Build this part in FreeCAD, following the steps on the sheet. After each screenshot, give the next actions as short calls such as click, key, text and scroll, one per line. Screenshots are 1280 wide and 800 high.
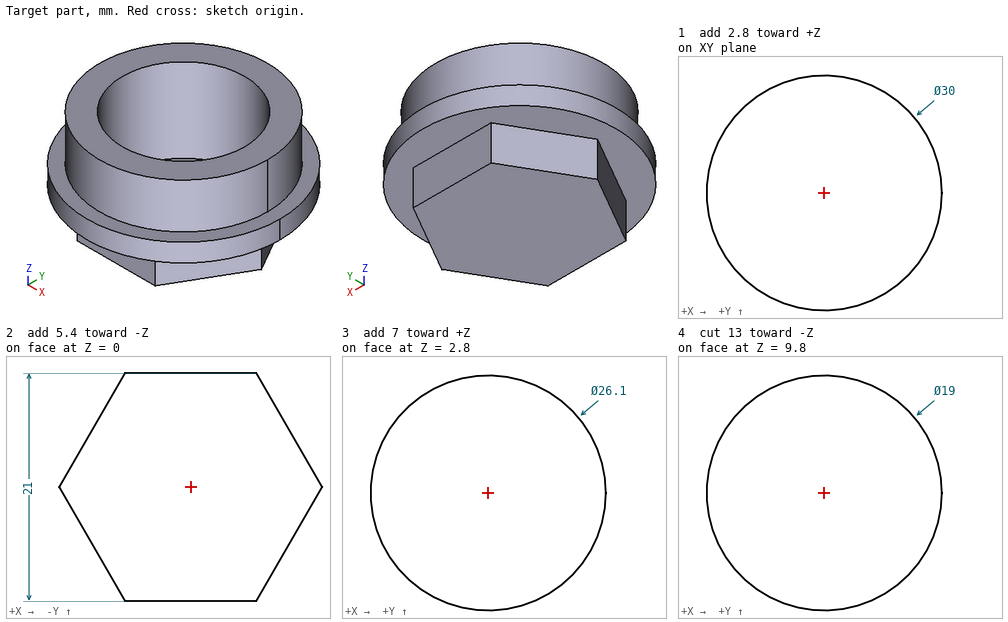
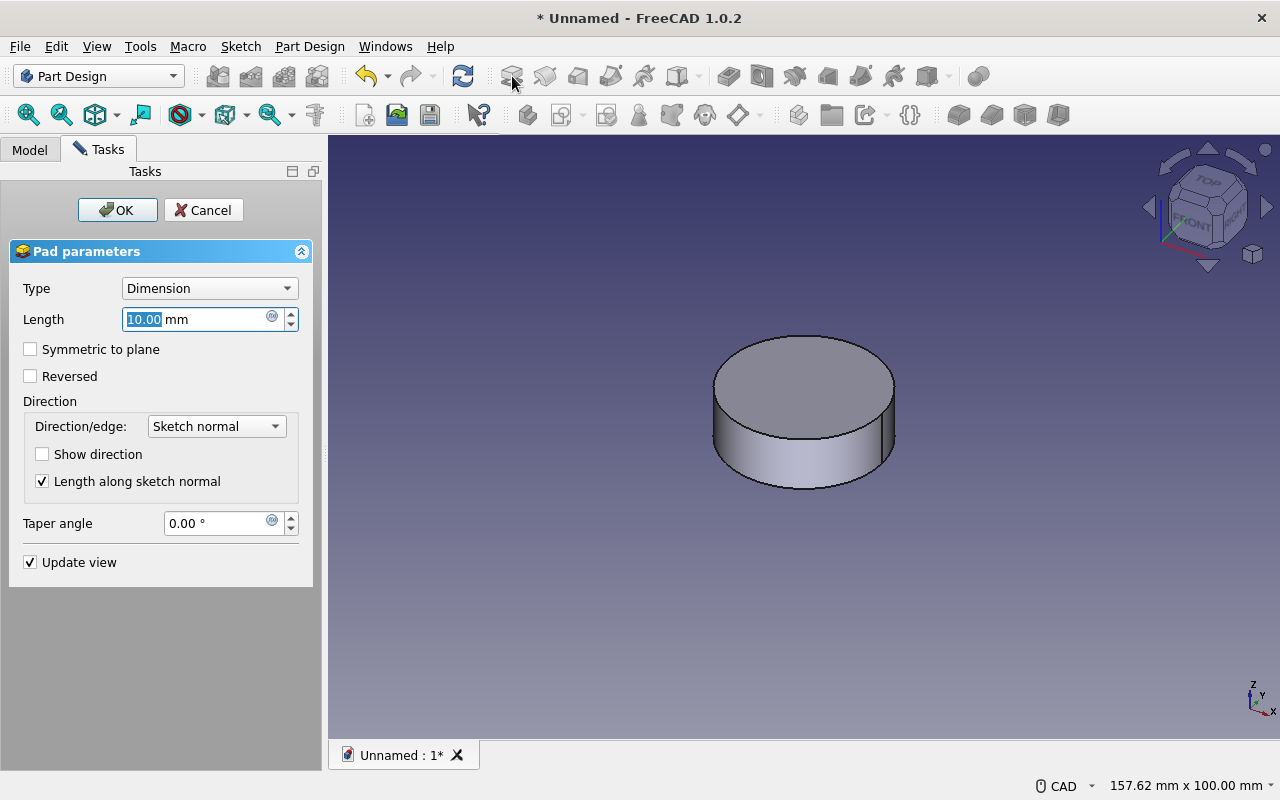
text(2.8)
key(Tab)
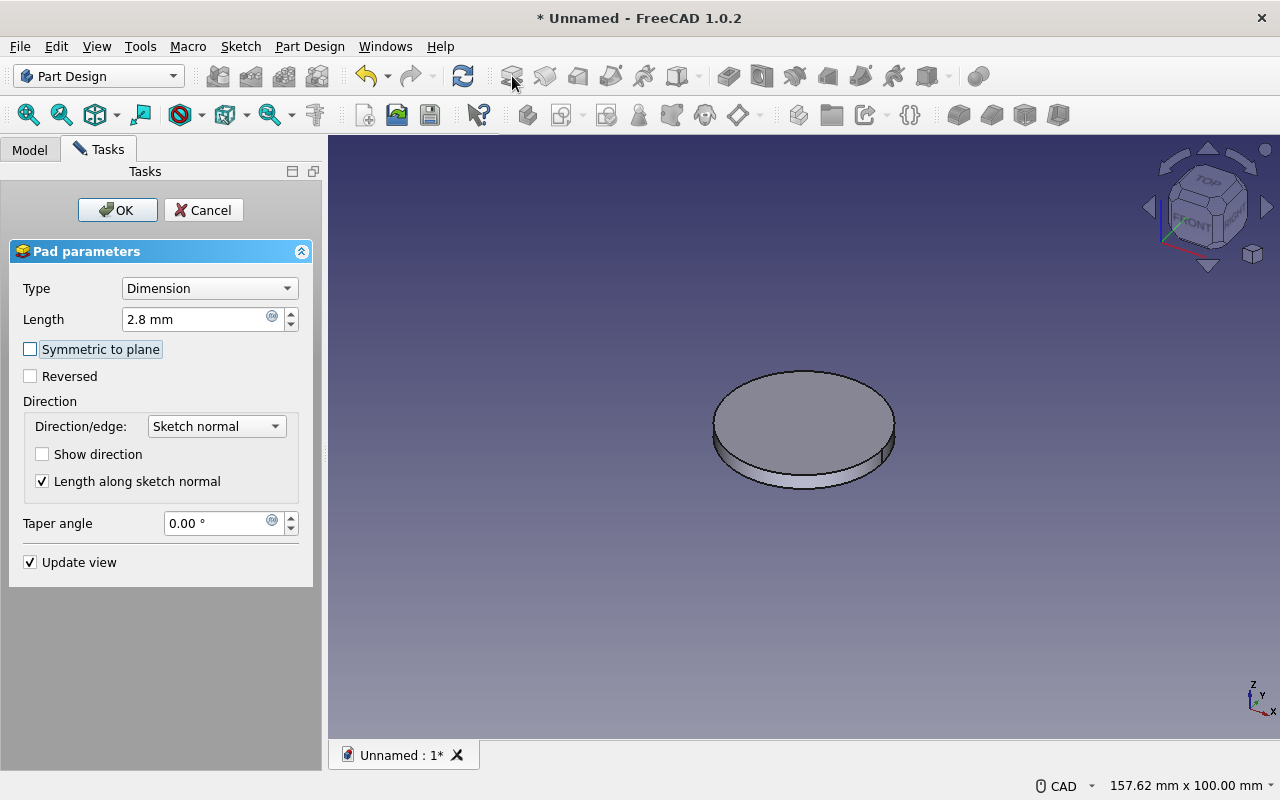
click(118, 210)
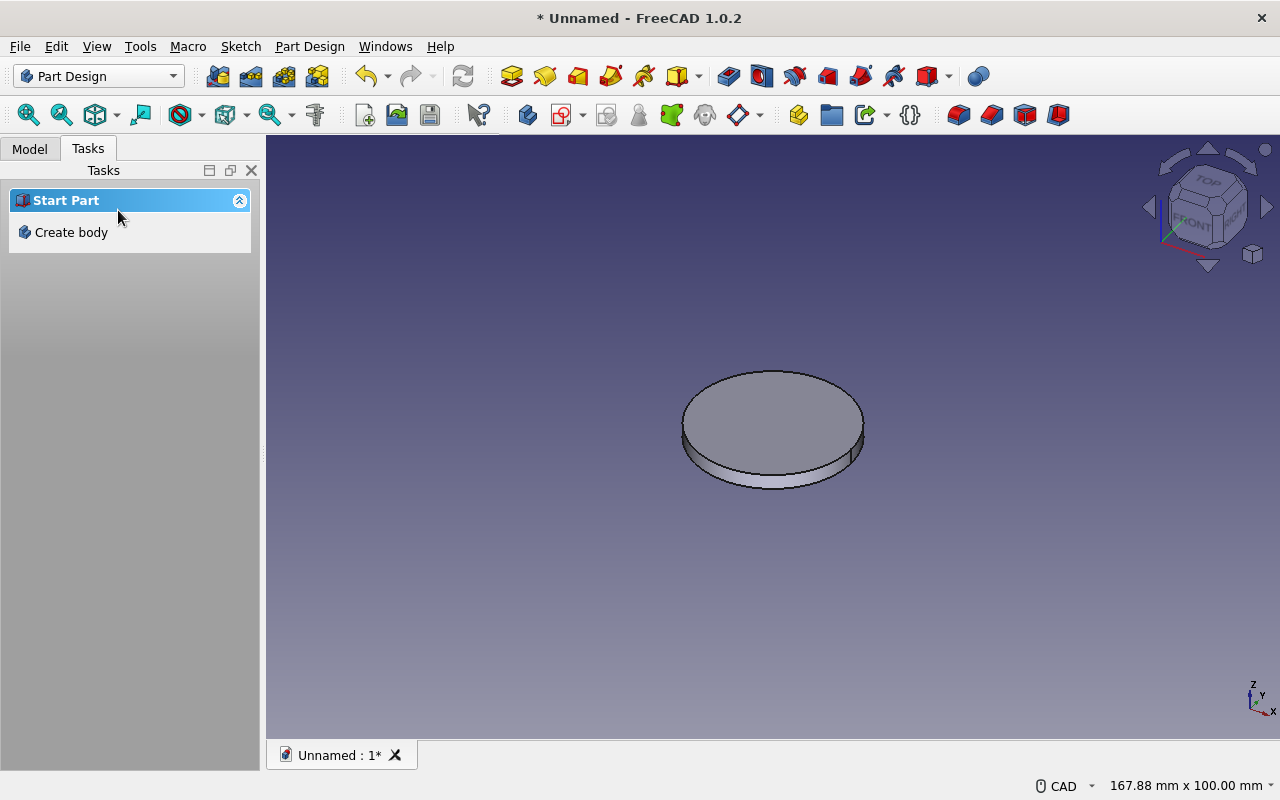
click(29, 116)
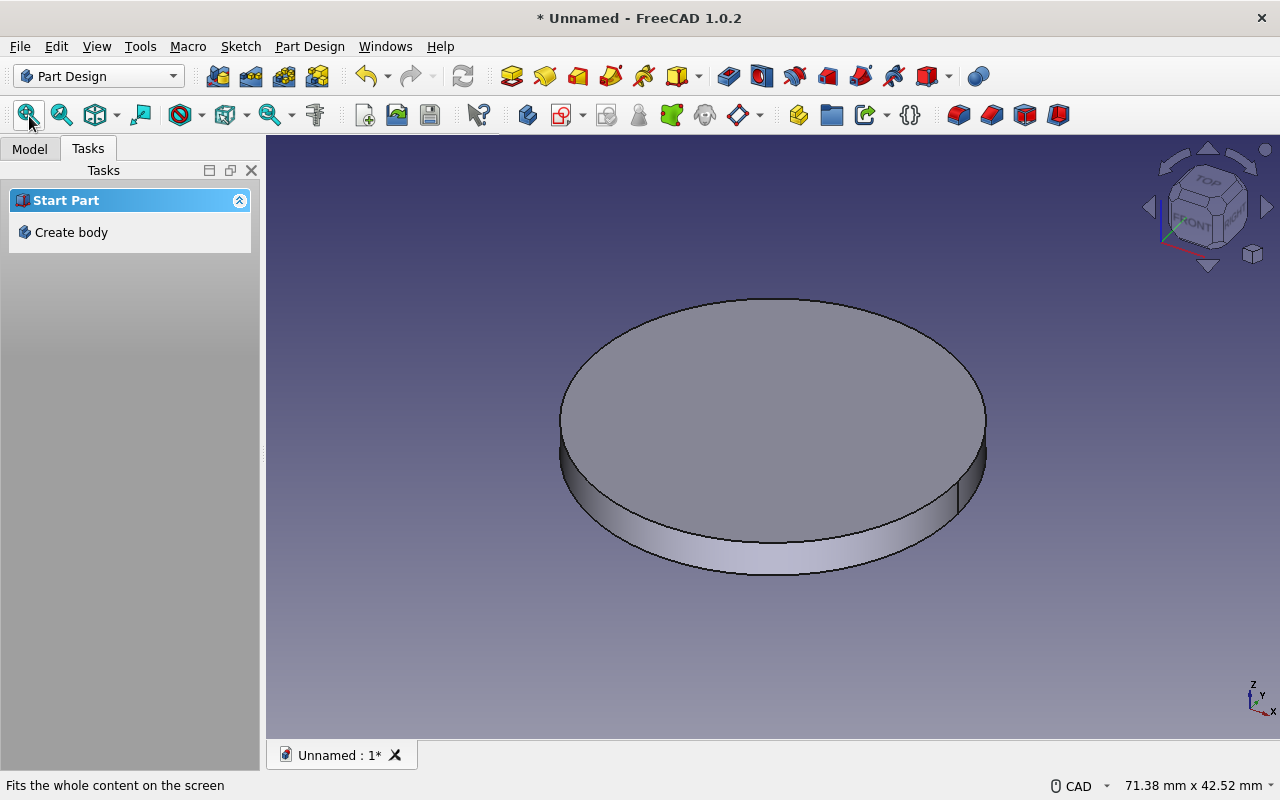
key(5)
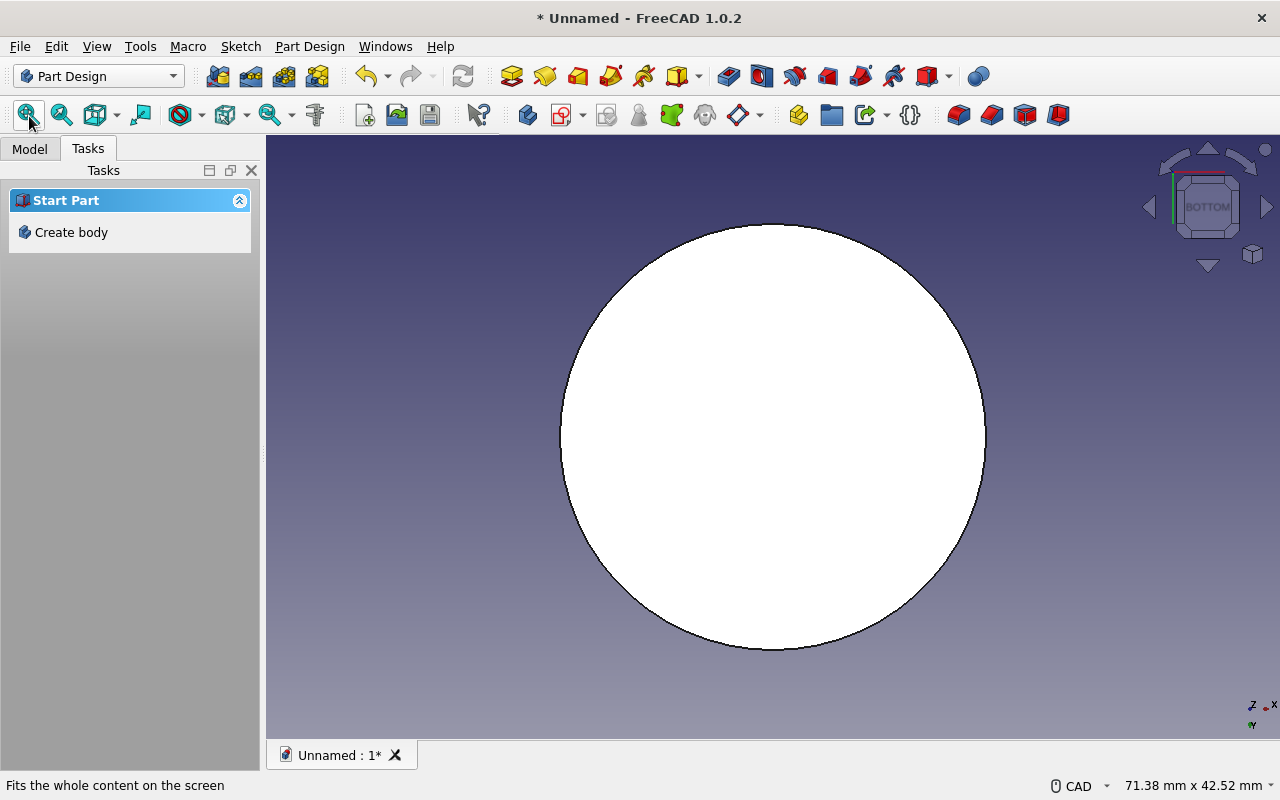
click(773, 436)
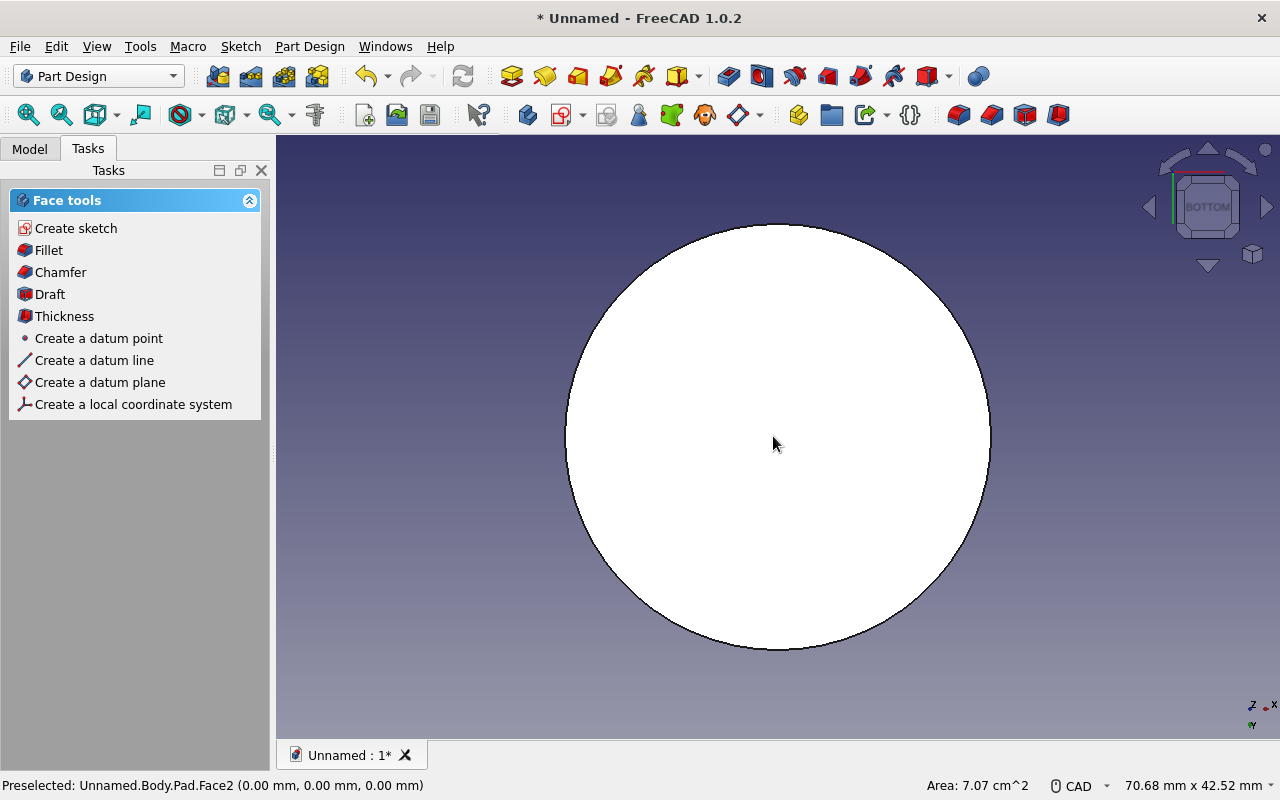
click(560, 116)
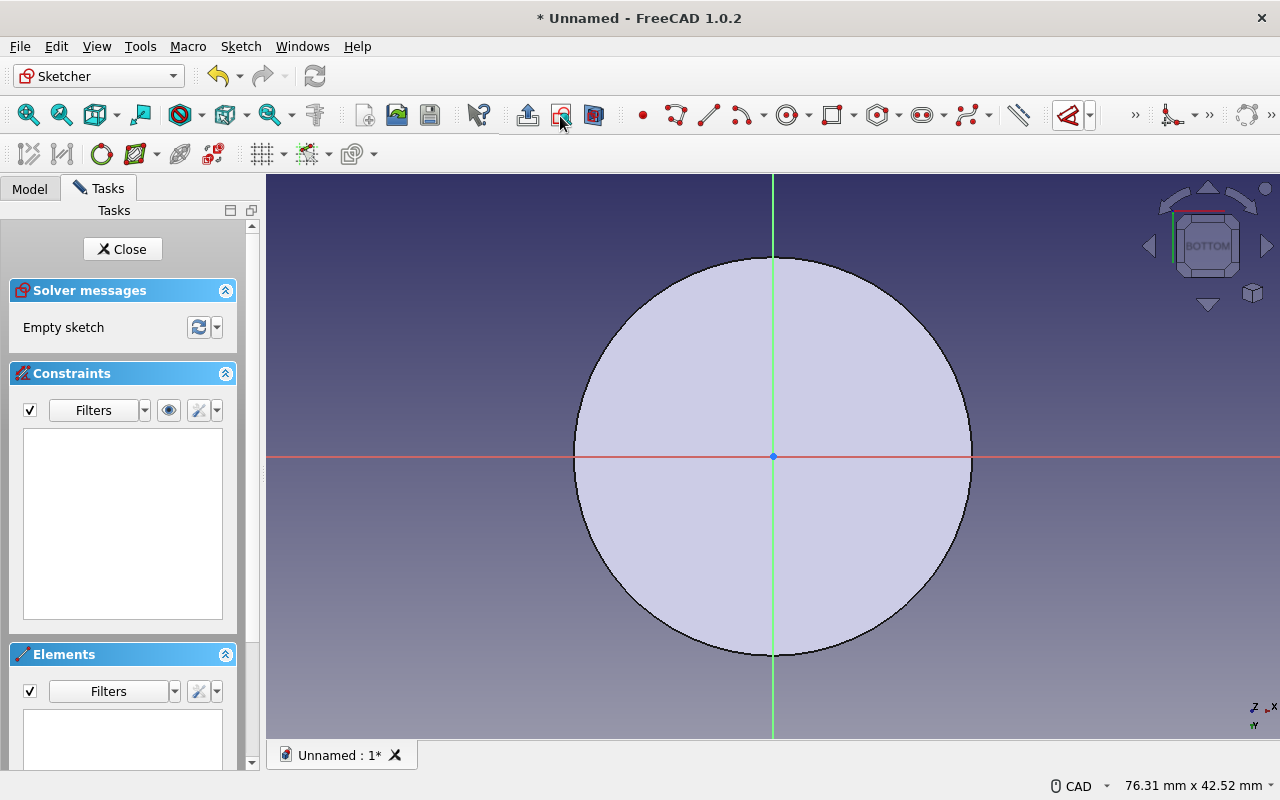
click(876, 116)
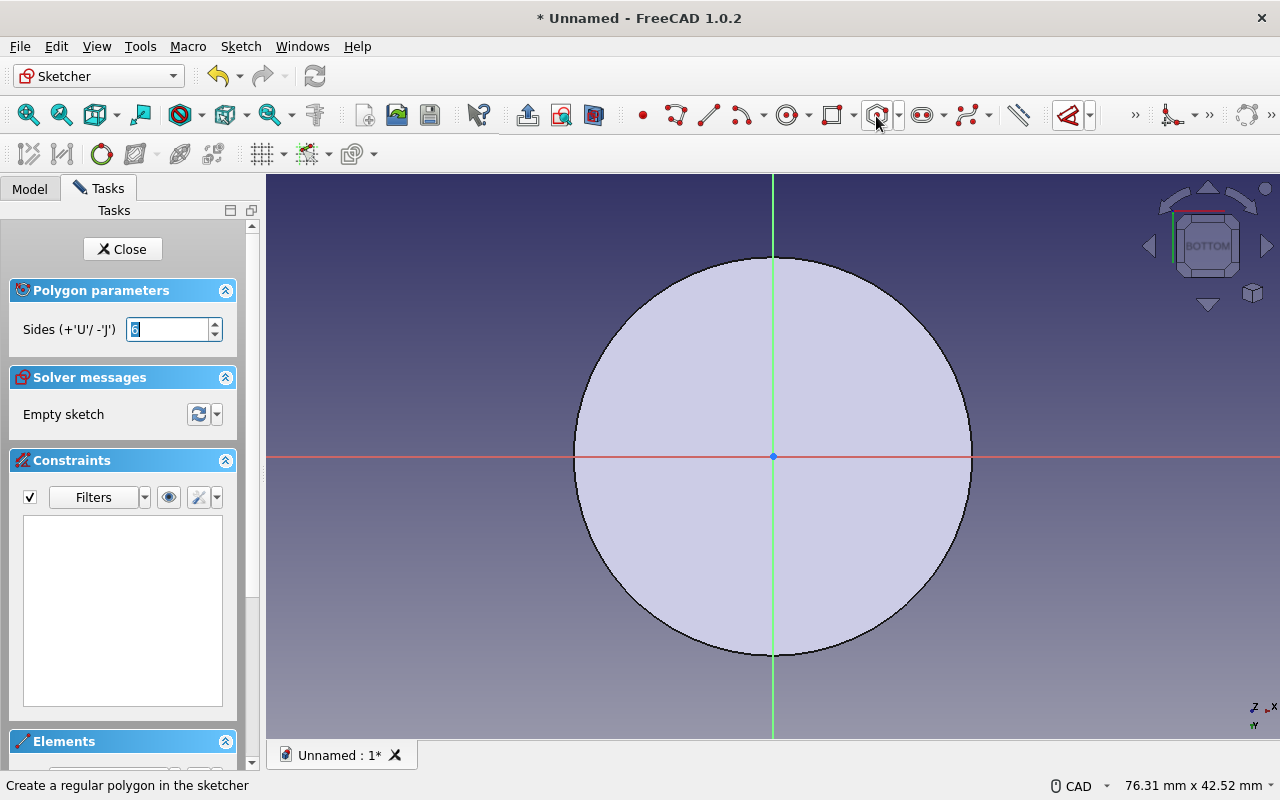
click(773, 456)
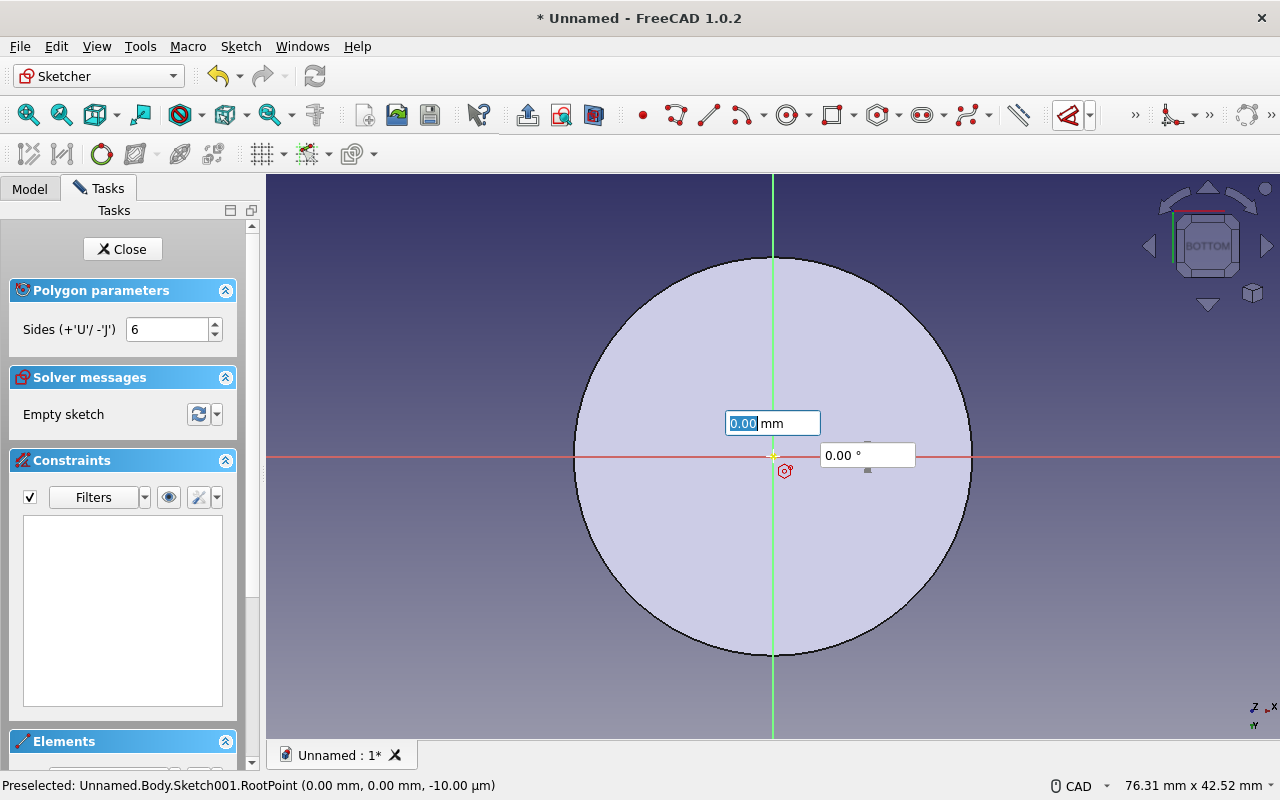
click(612, 456)
right_click(612, 456)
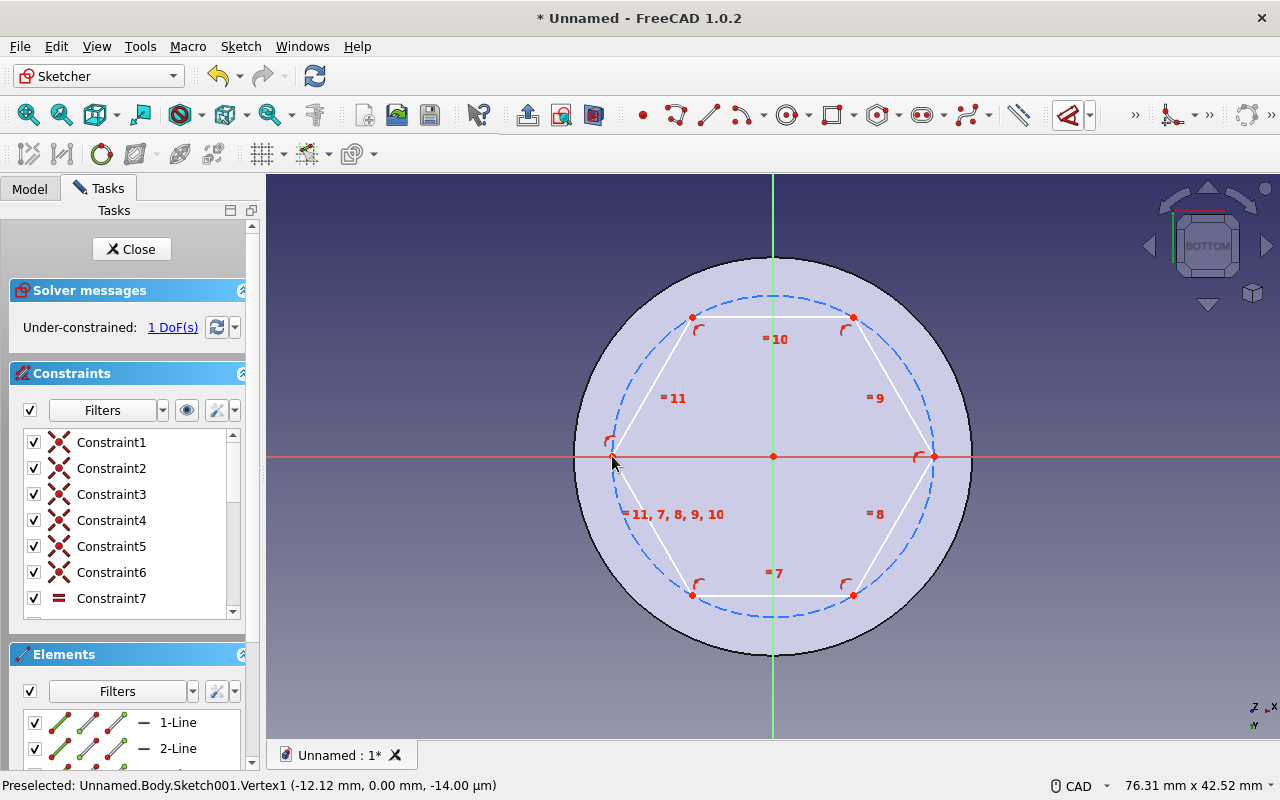
click(1068, 116)